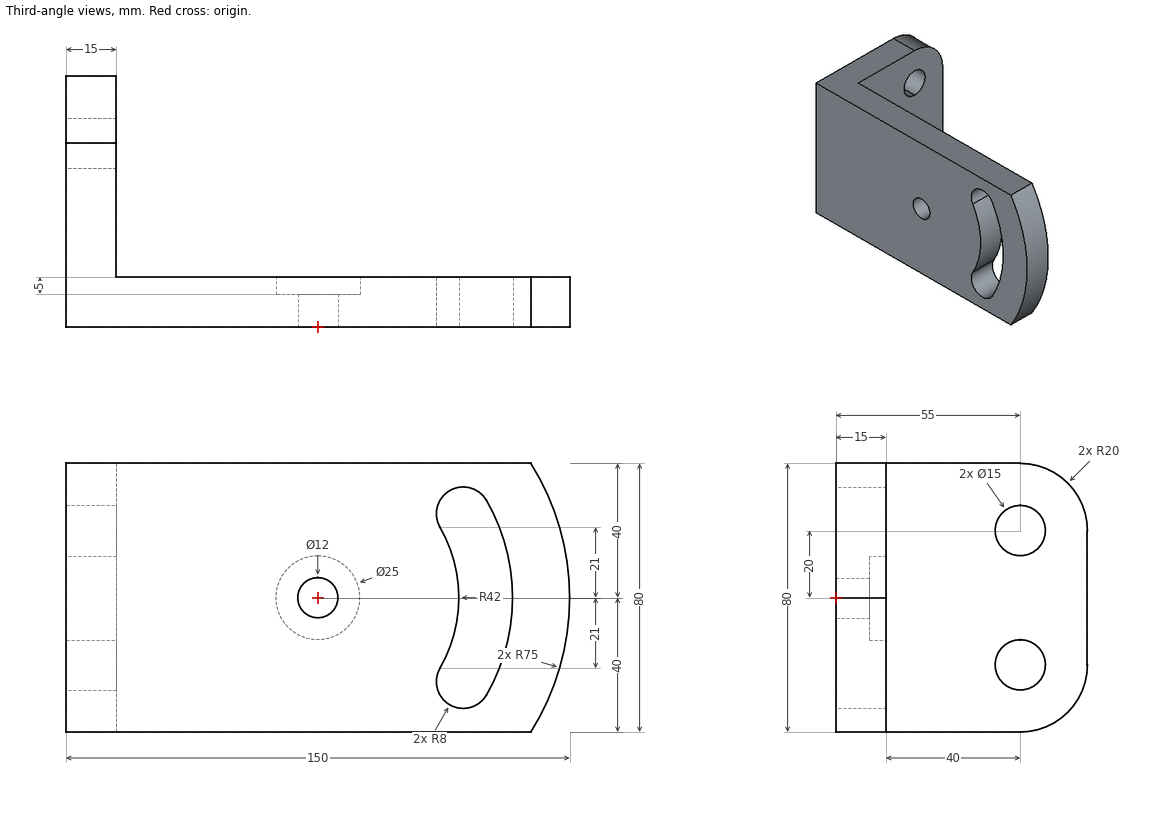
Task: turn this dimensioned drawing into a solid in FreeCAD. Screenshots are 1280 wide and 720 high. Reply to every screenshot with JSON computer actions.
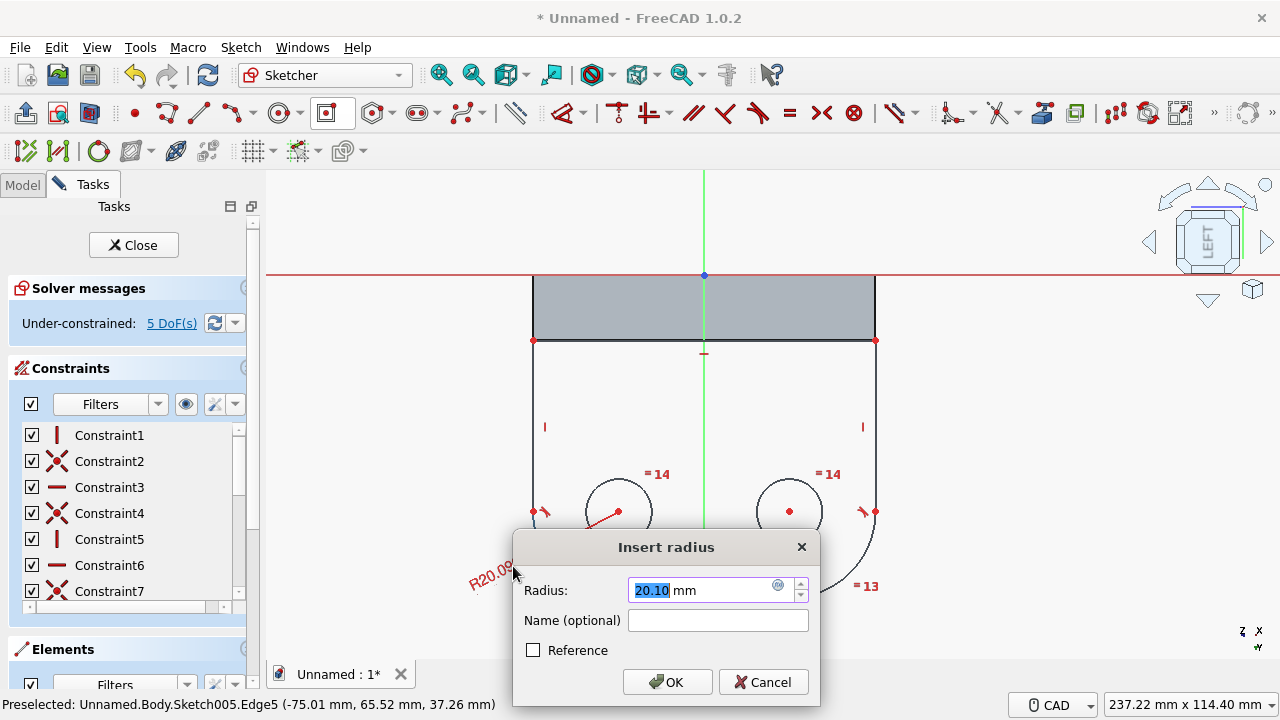
{"action": "type", "text": "20"}
{"action": "key", "text": "Return"}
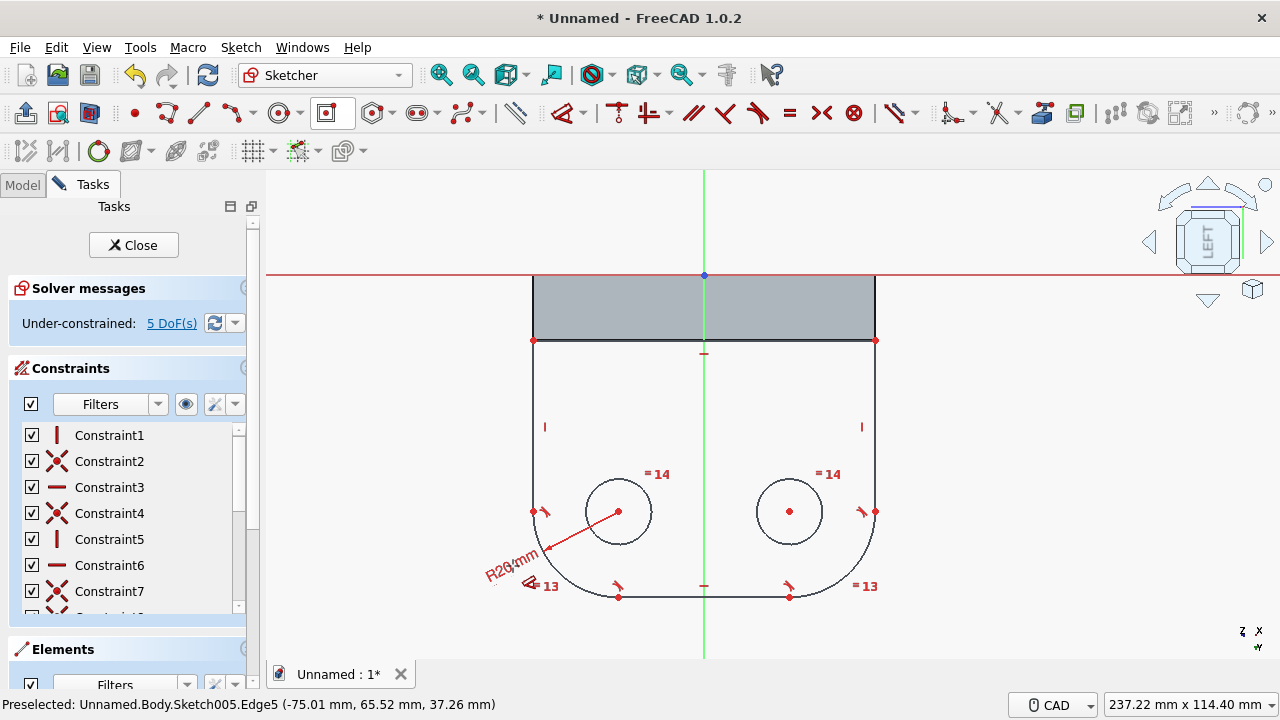
{"action": "left_click", "coordinate": [642, 489]}
{"action": "left_click", "coordinate": [665, 467]}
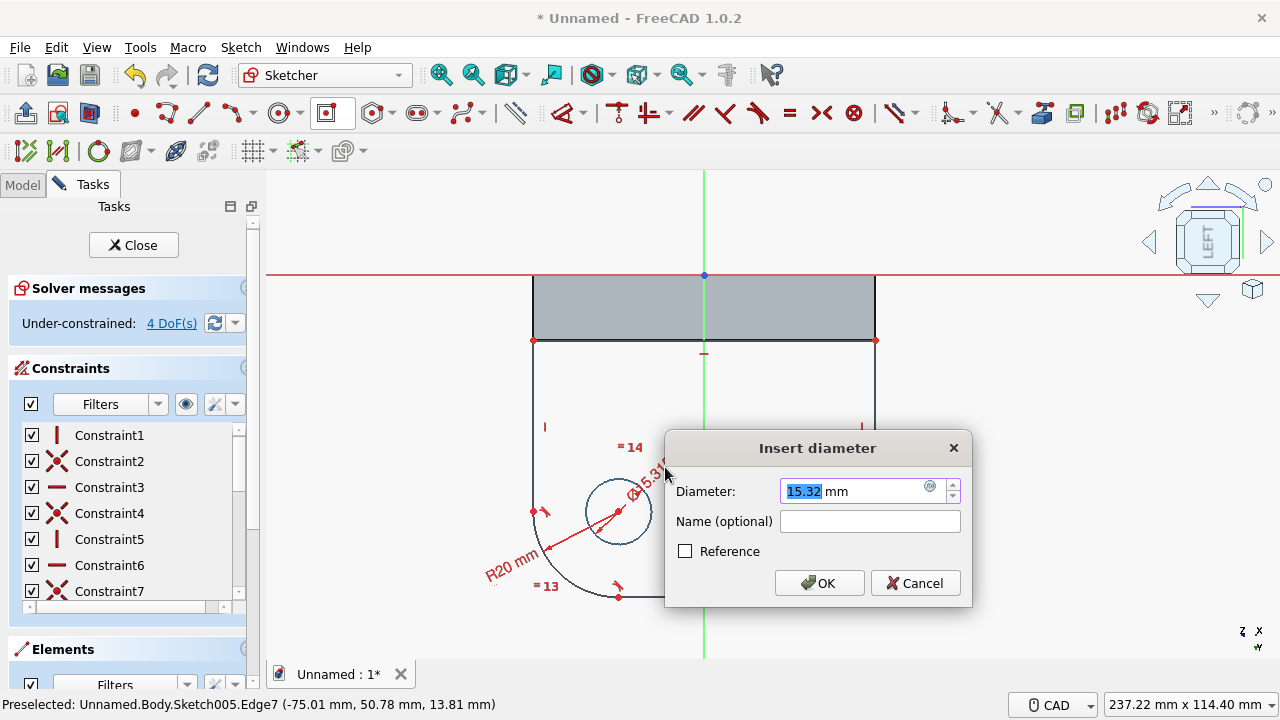
{"action": "type", "text": "15"}
{"action": "key", "text": "Return"}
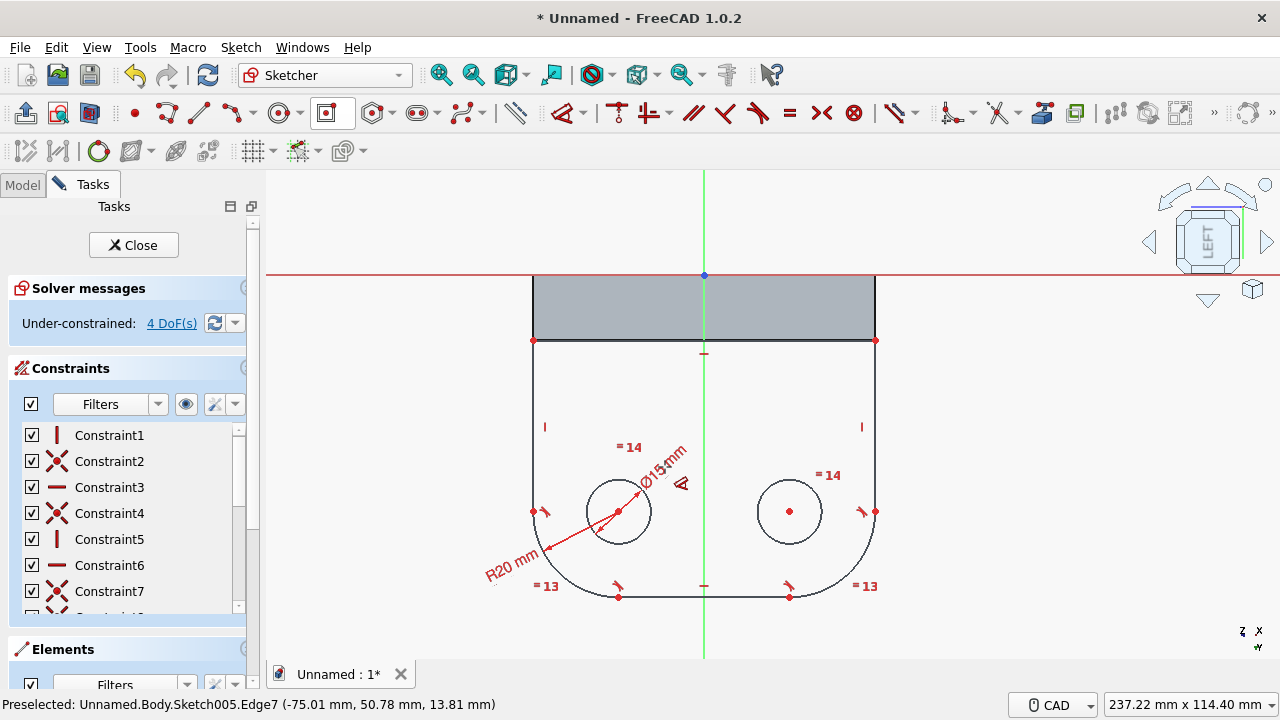
{"action": "left_click", "coordinate": [875, 461]}
{"action": "left_click", "coordinate": [909, 426]}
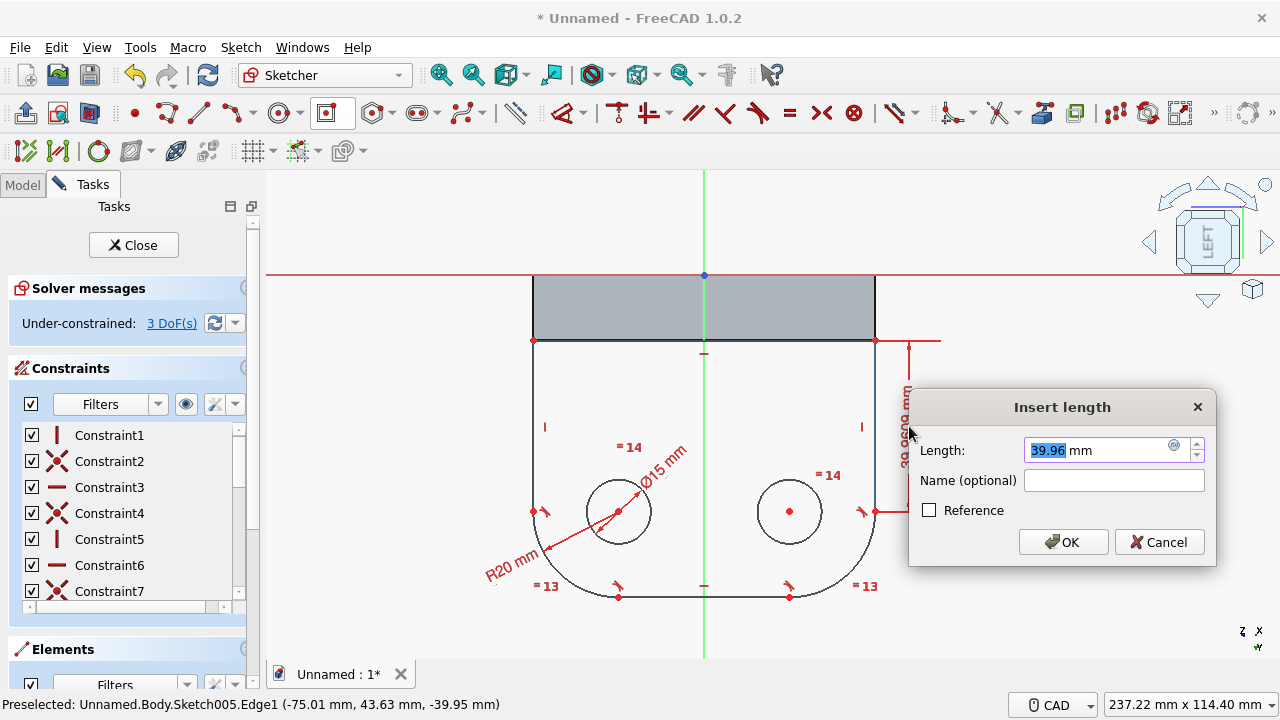
{"action": "type", "text": "40"}
{"action": "key", "text": "Return"}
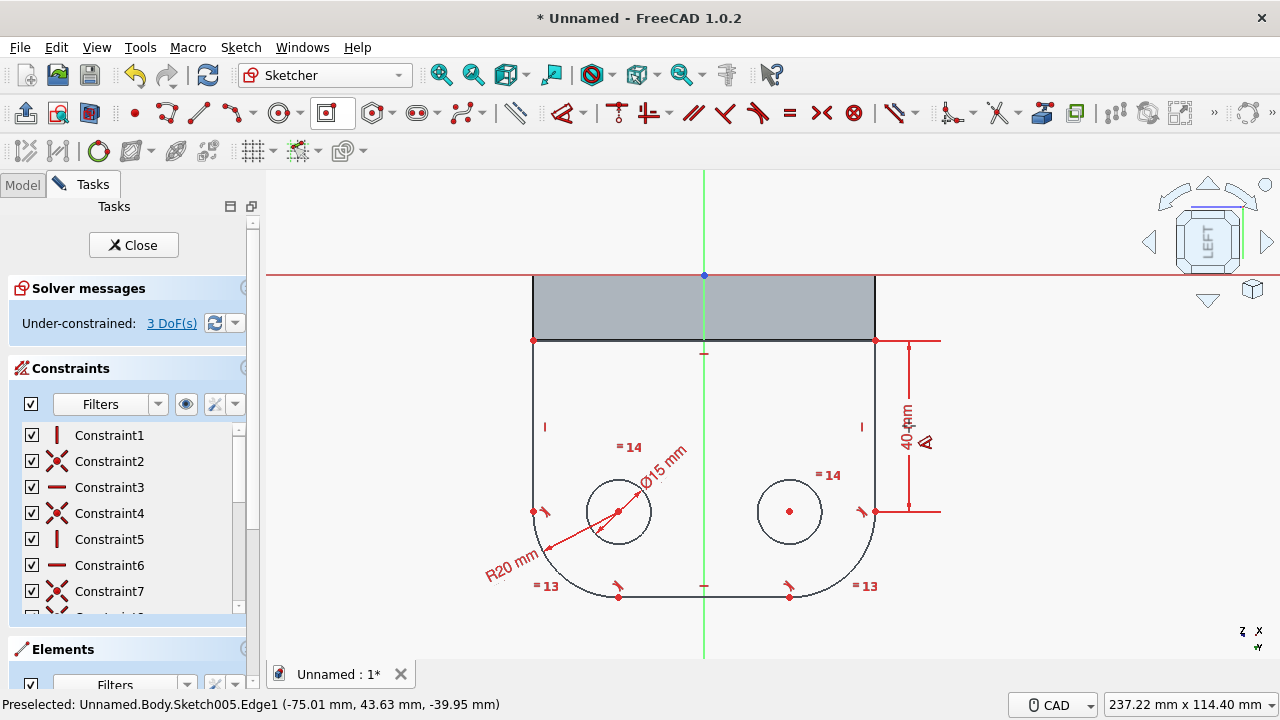
{"action": "left_click", "coordinate": [773, 341]}
{"action": "left_click", "coordinate": [626, 307]}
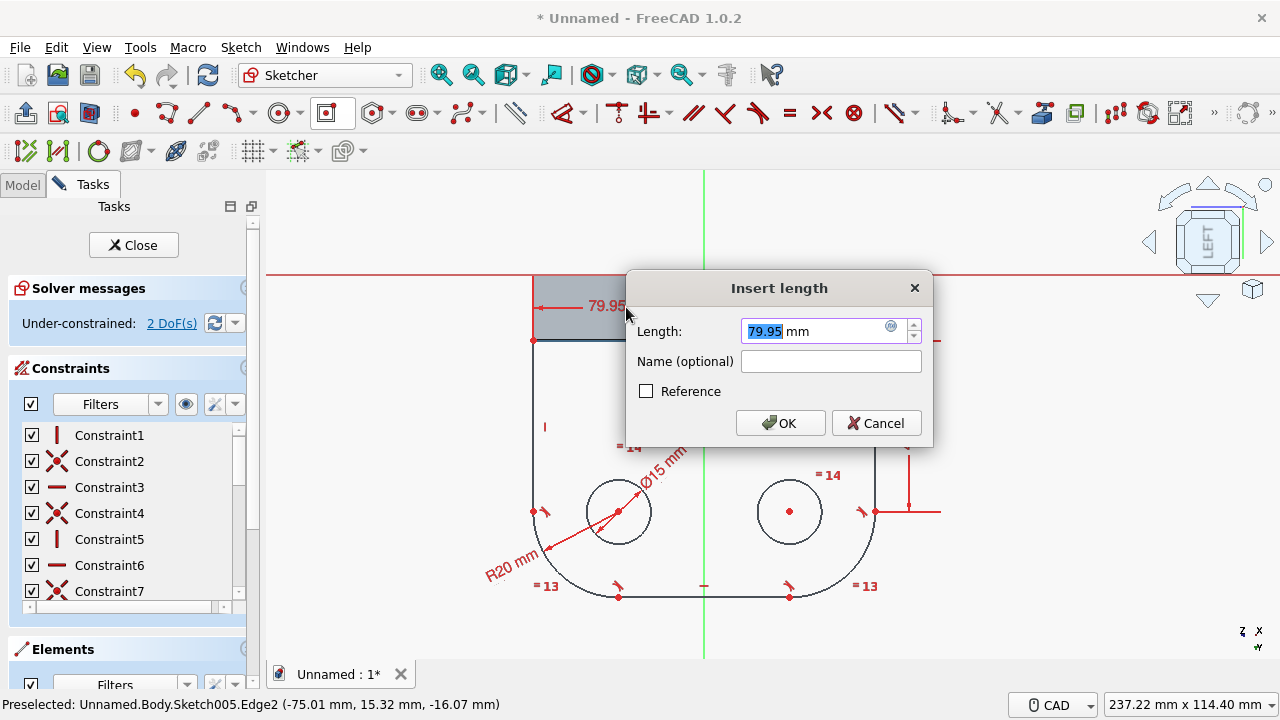
{"action": "type", "text": "80"}
{"action": "key", "text": "Return"}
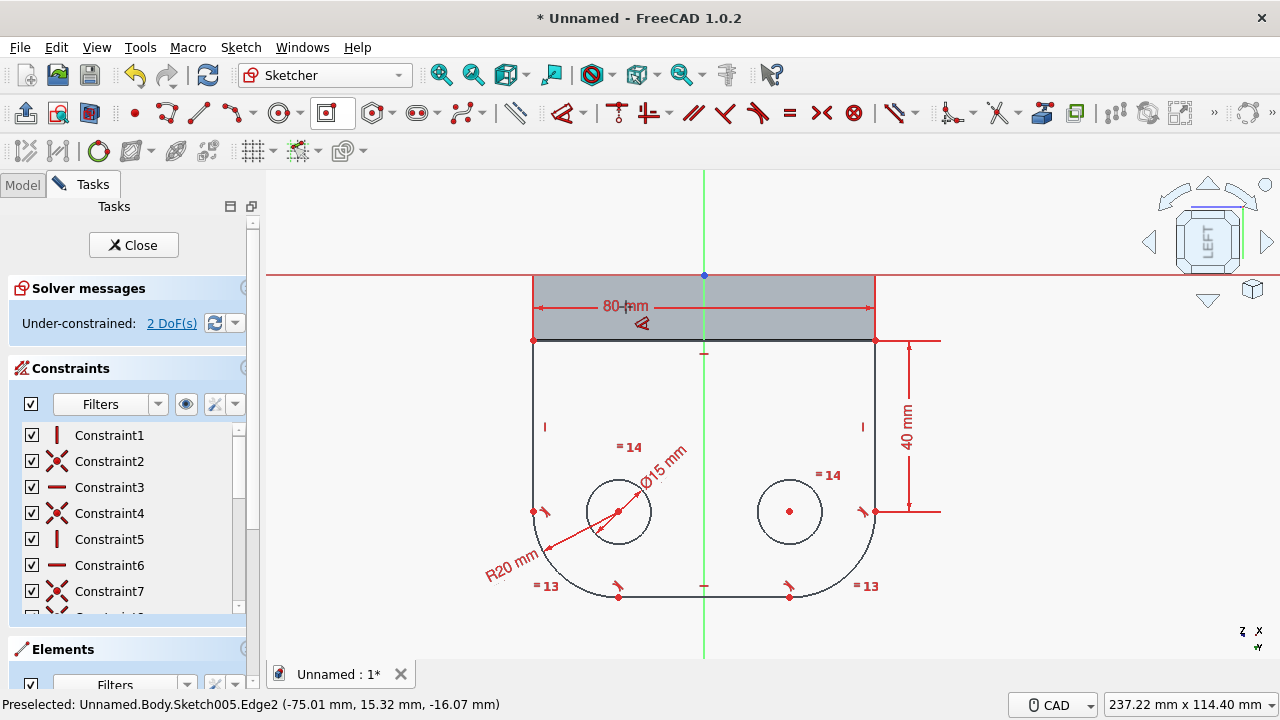
{"action": "left_click", "coordinate": [619, 512]}
{"action": "left_click", "coordinate": [662, 241]}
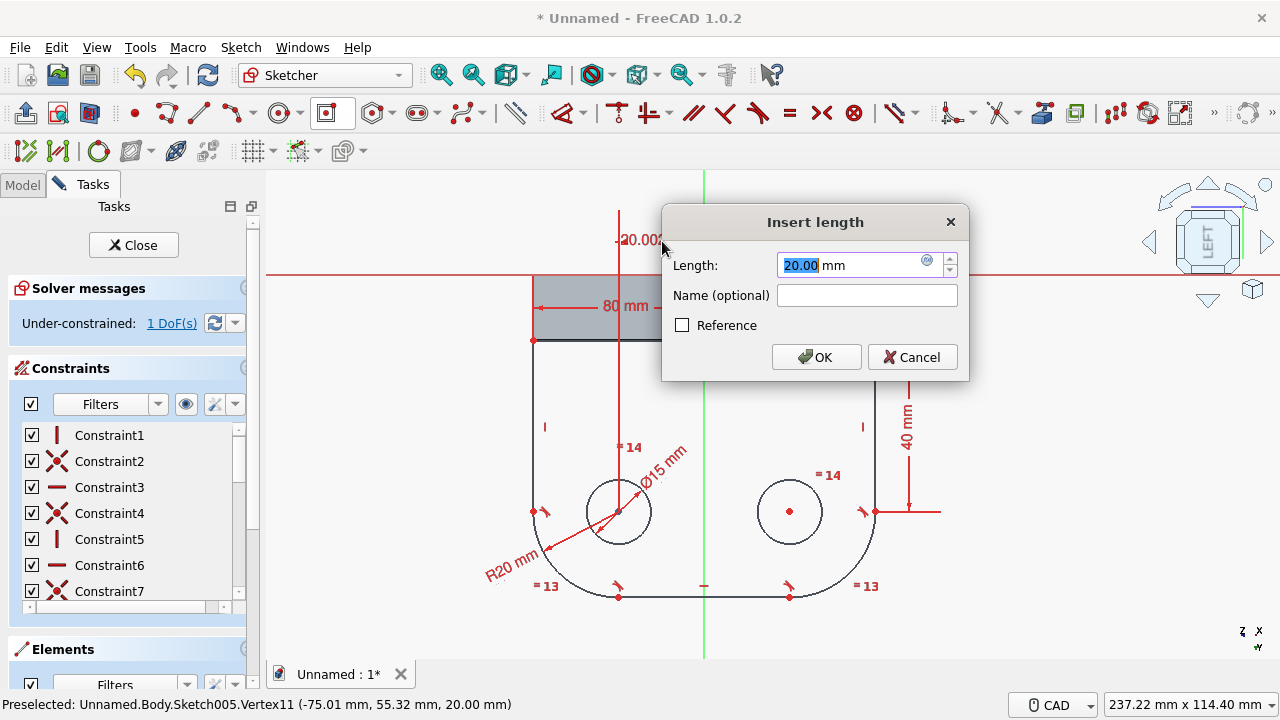
{"action": "type", "text": "20"}
{"action": "key", "text": "Return"}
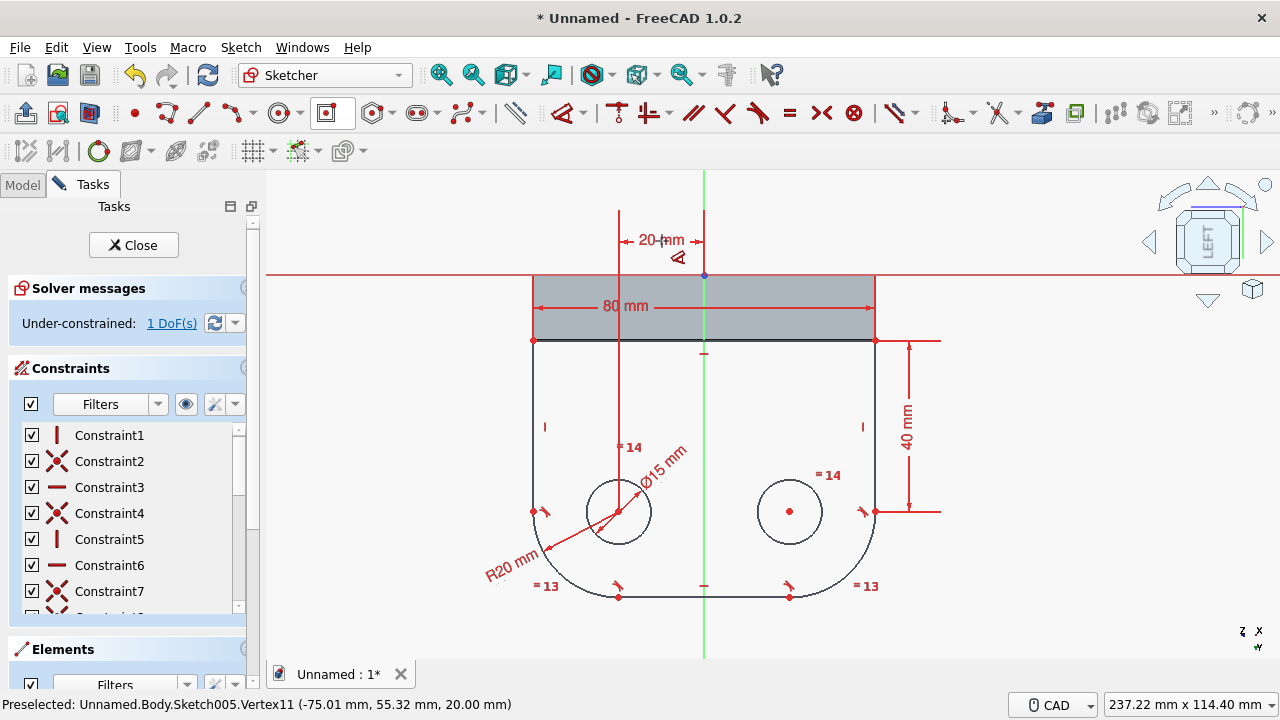
{"action": "left_click", "coordinate": [619, 512]}
{"action": "left_click", "coordinate": [585, 394]}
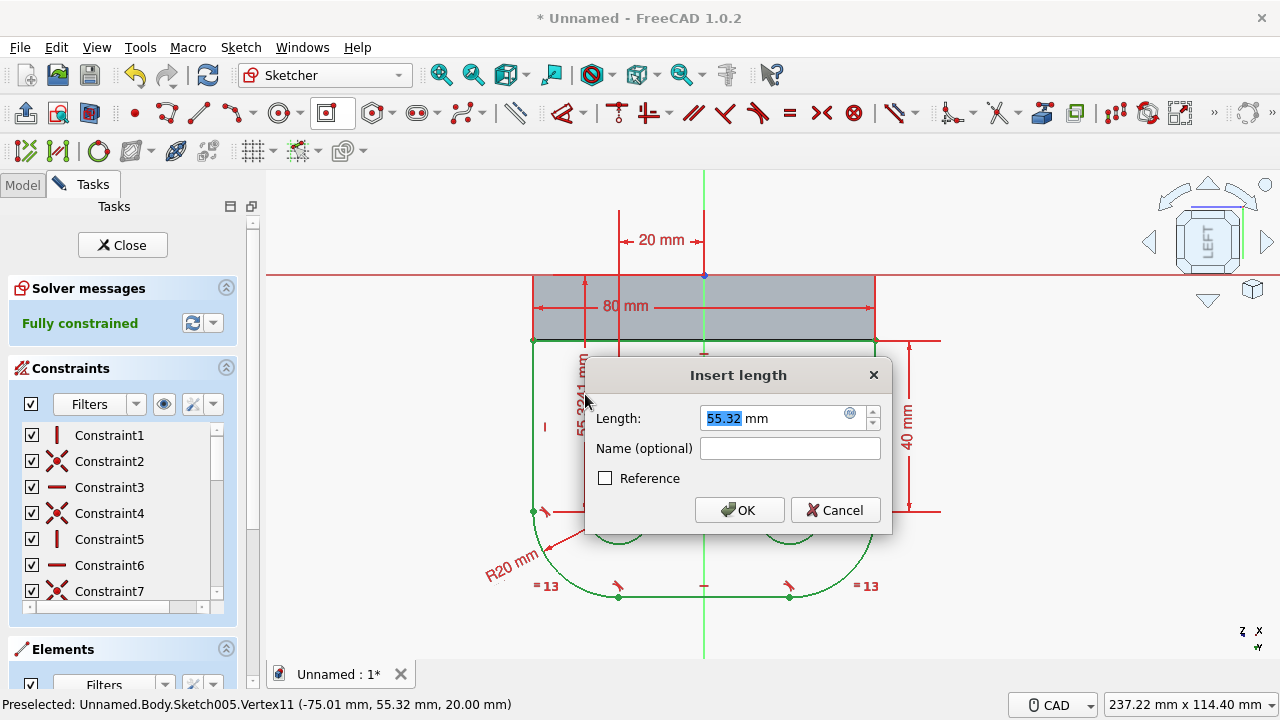
{"action": "type", "text": "55"}
{"action": "key", "text": "Return"}
{"action": "key", "text": "Escape"}